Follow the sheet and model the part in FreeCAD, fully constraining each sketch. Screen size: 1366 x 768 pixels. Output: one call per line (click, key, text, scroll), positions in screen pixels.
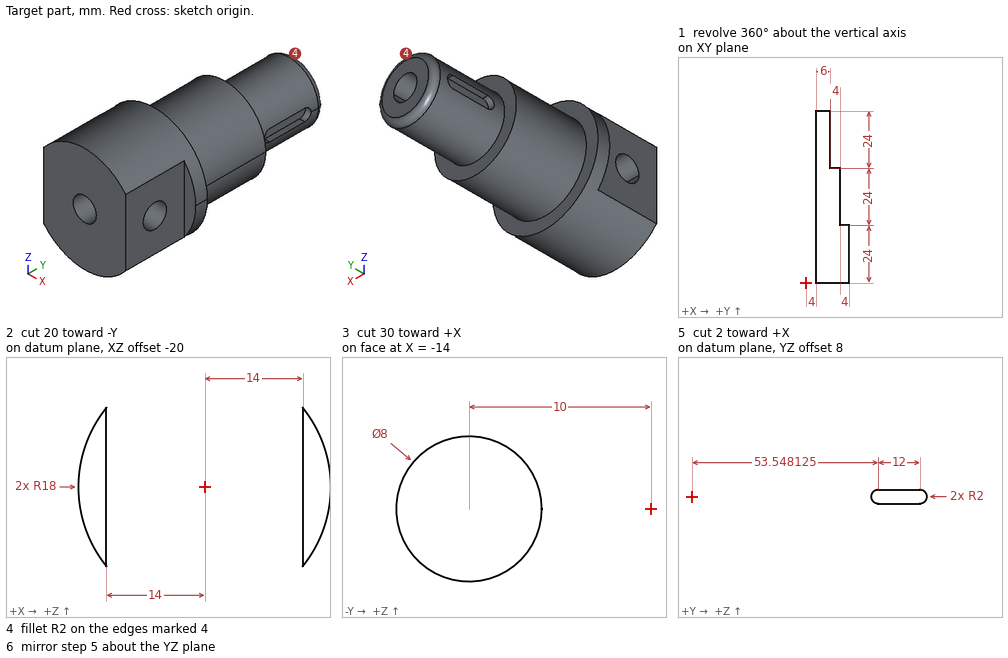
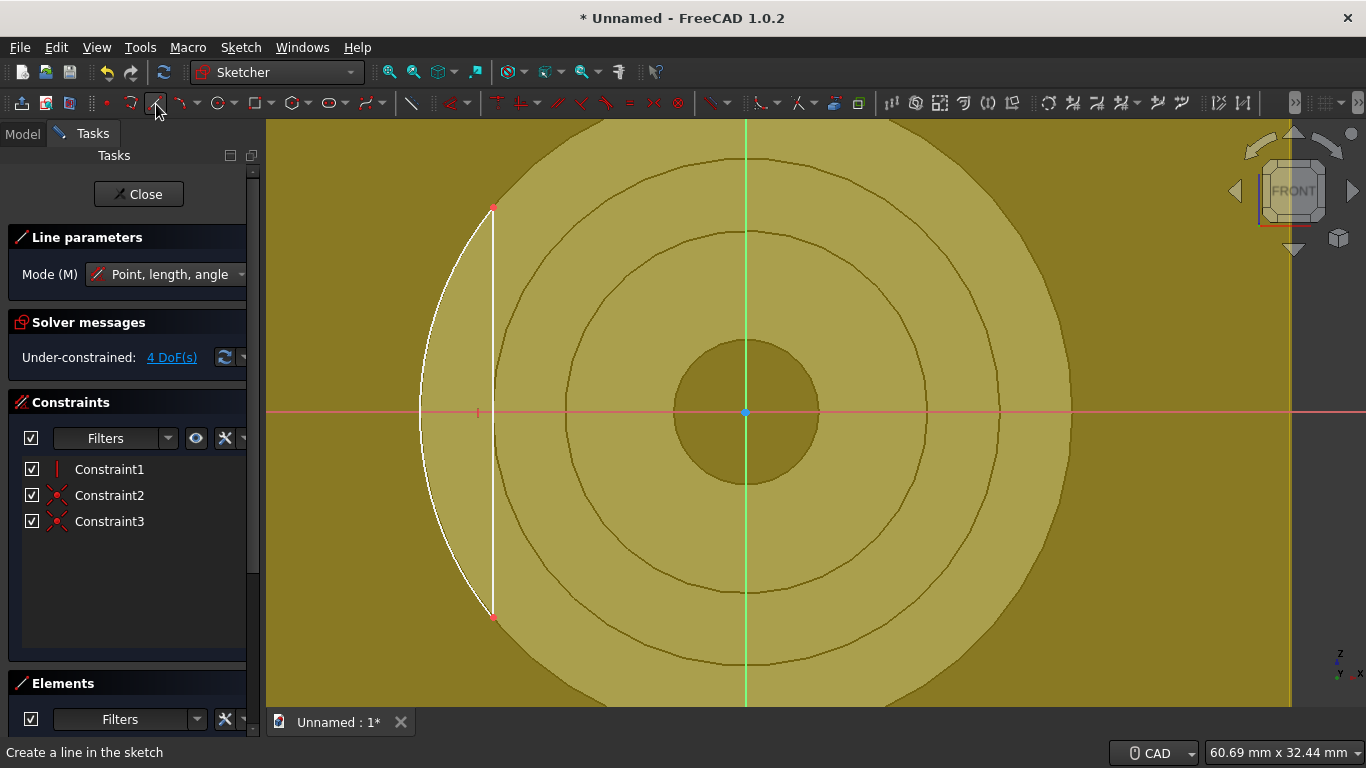
click(1000, 207)
click(1000, 617)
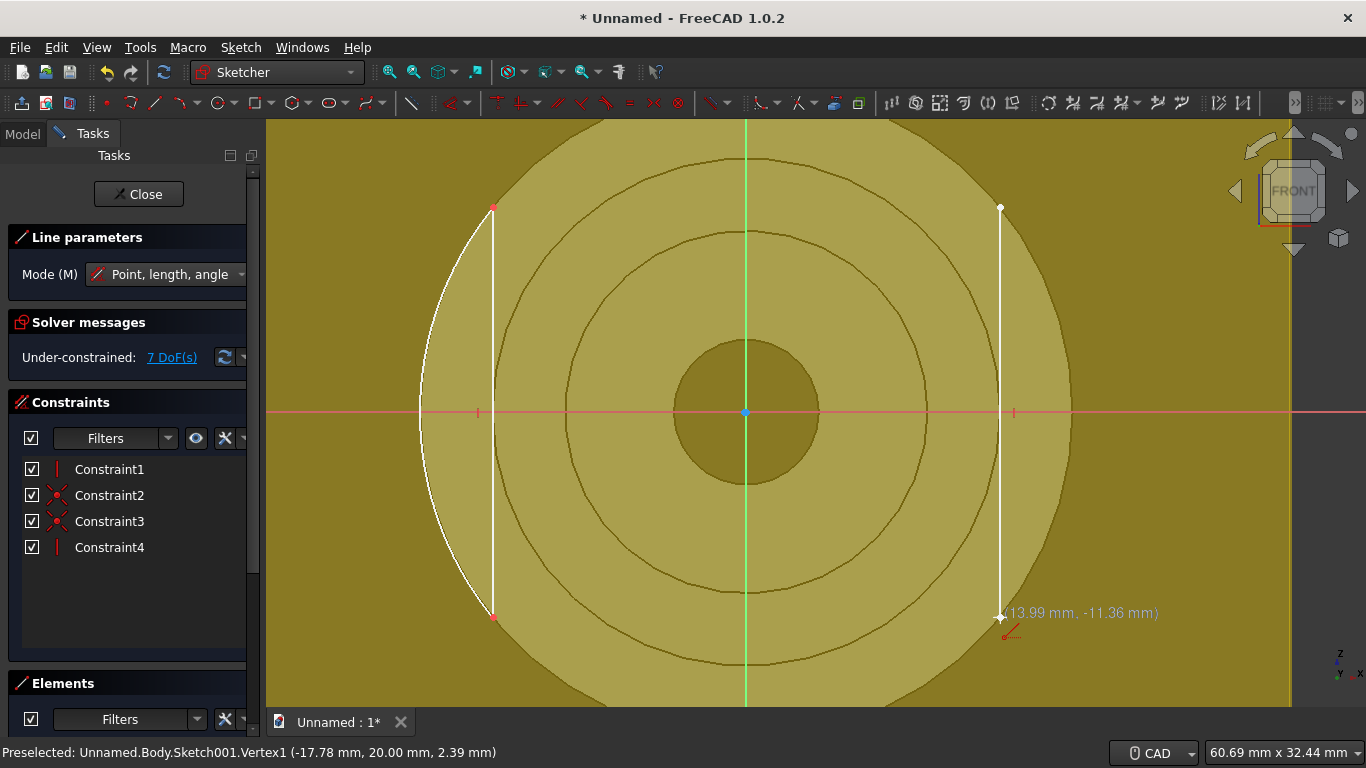
click(180, 104)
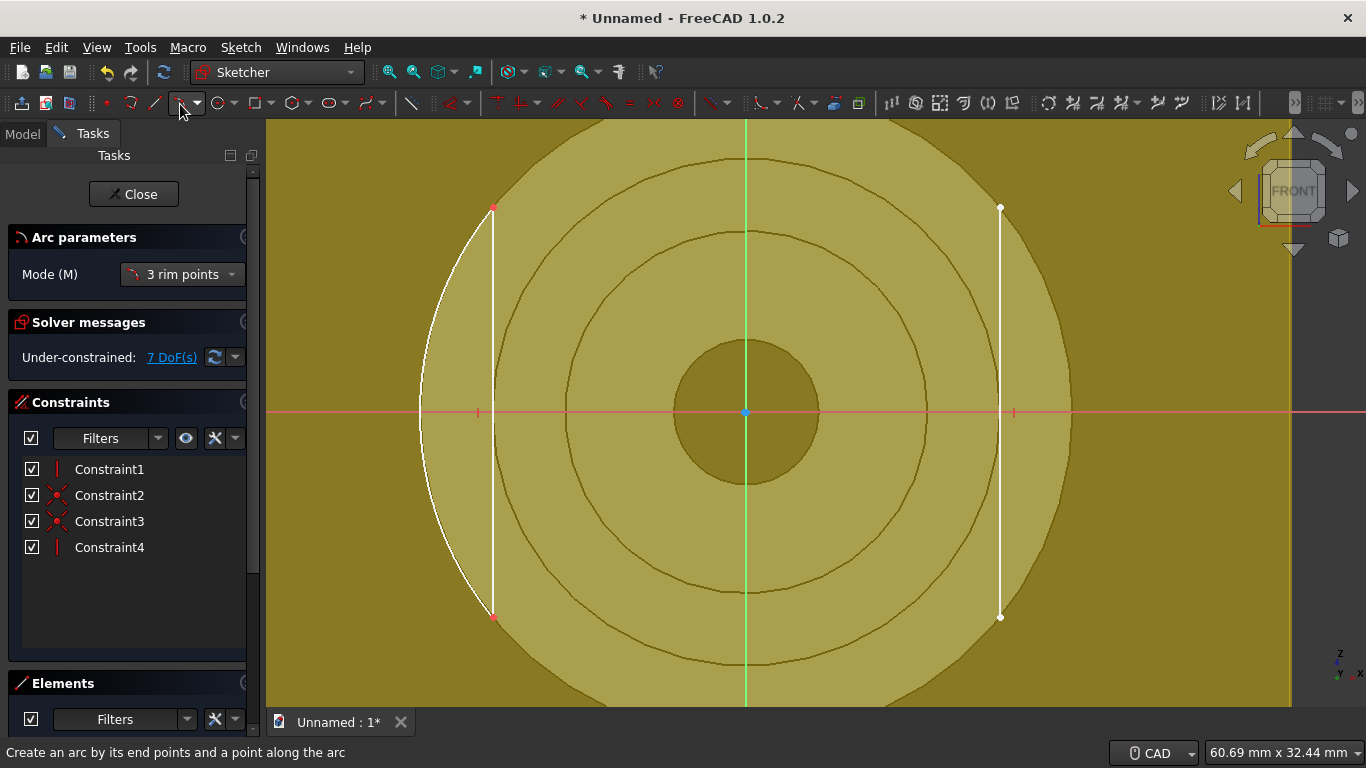
click(1000, 618)
click(1000, 208)
click(1070, 456)
key(Escape)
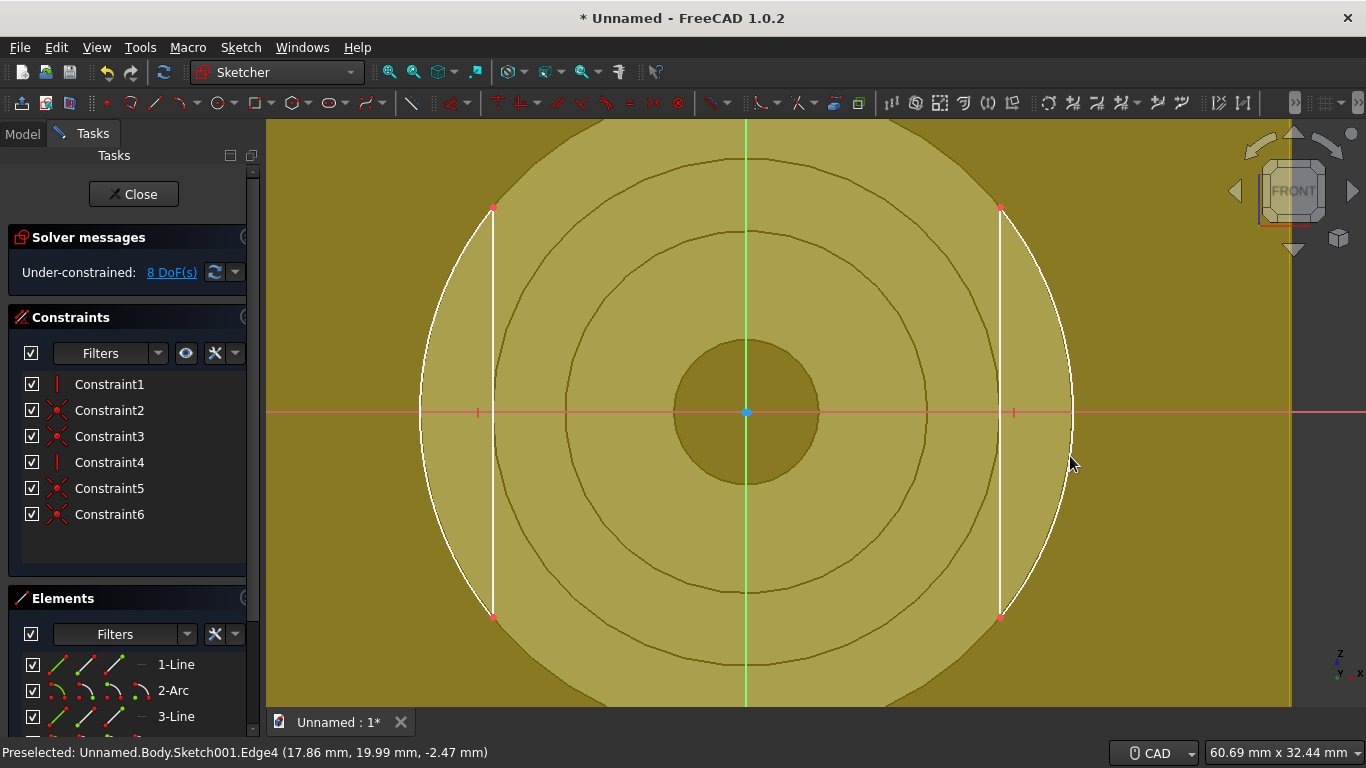
click(432, 325)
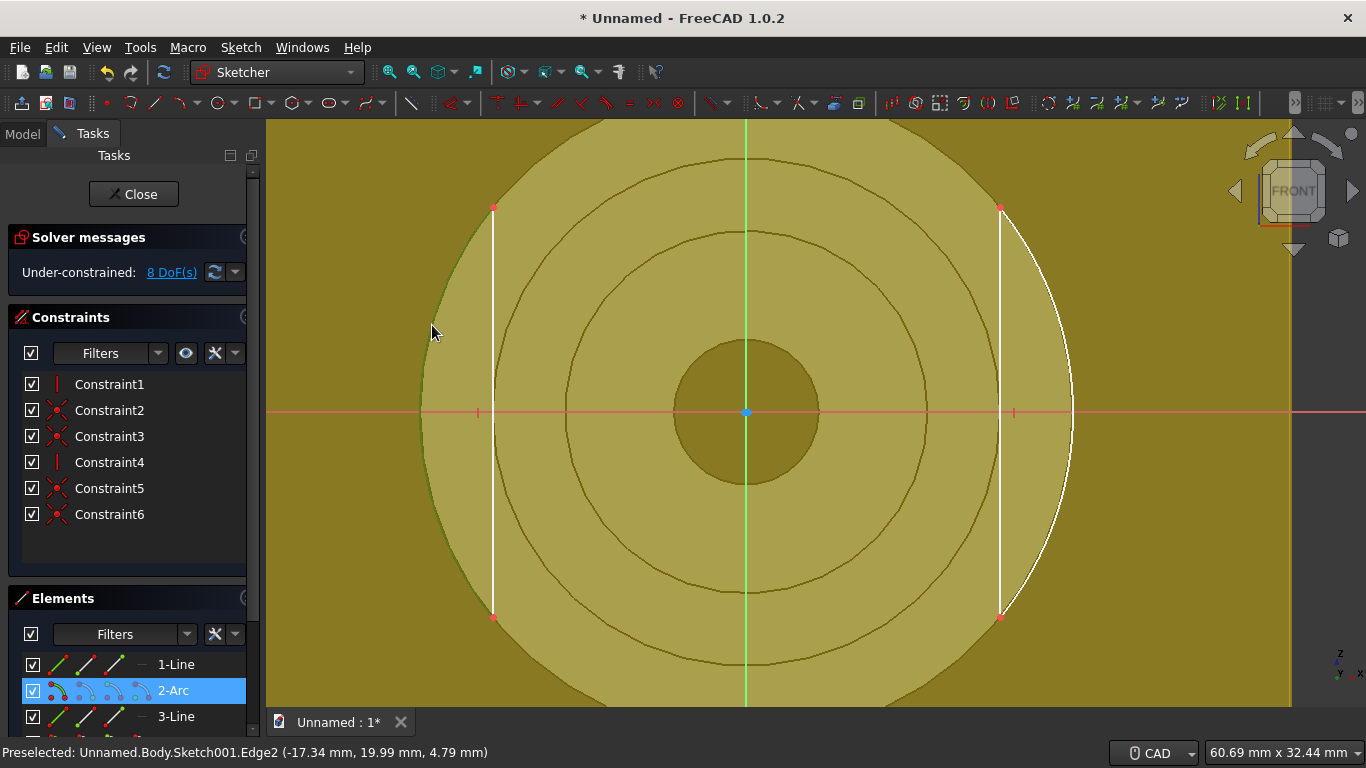
click(1061, 501)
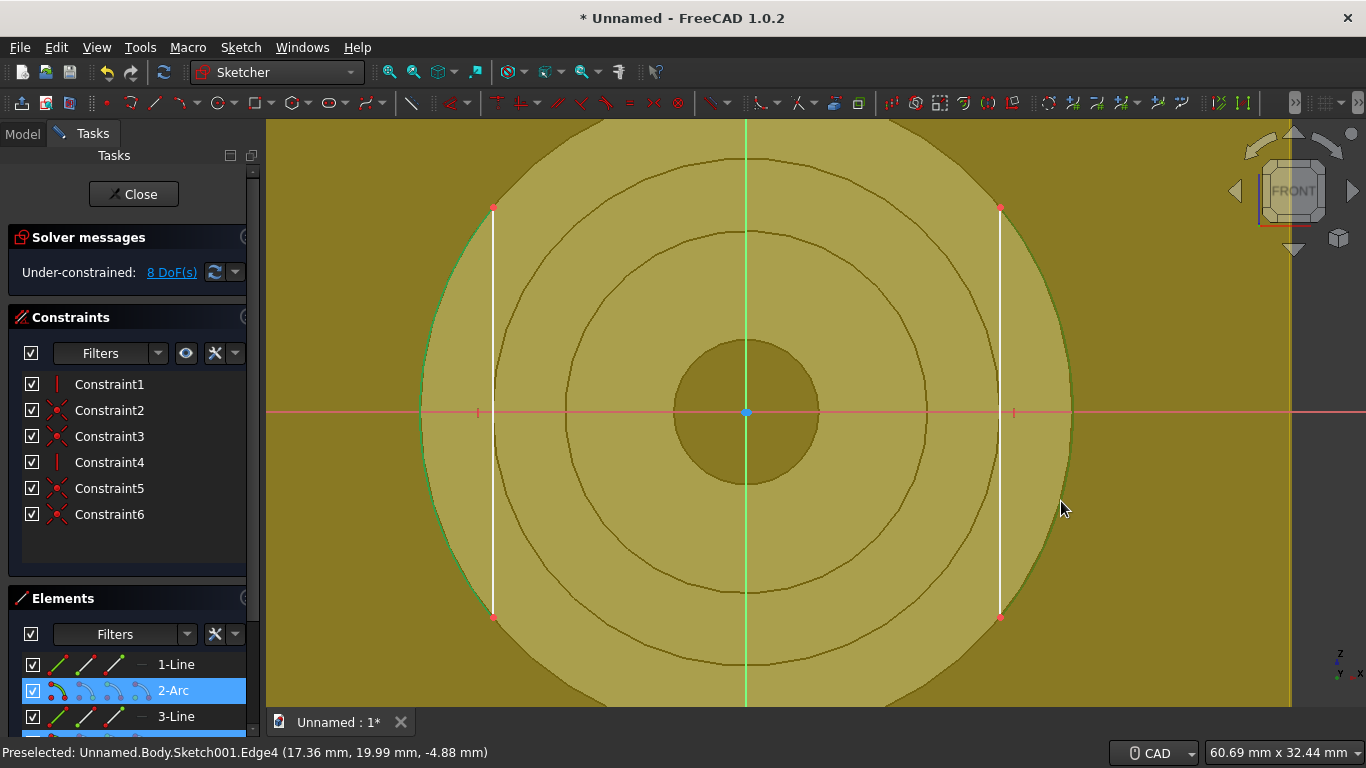
click(498, 104)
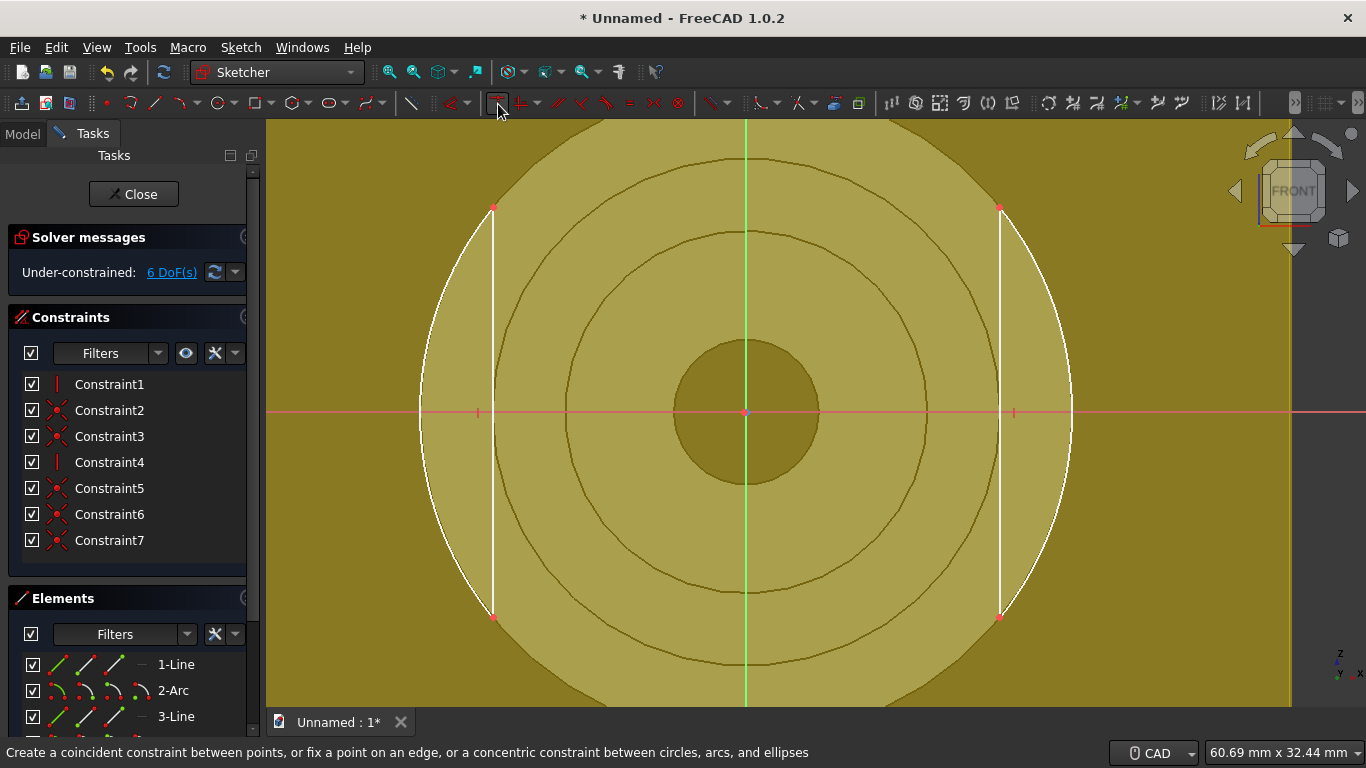
drag(734, 402, 756, 423)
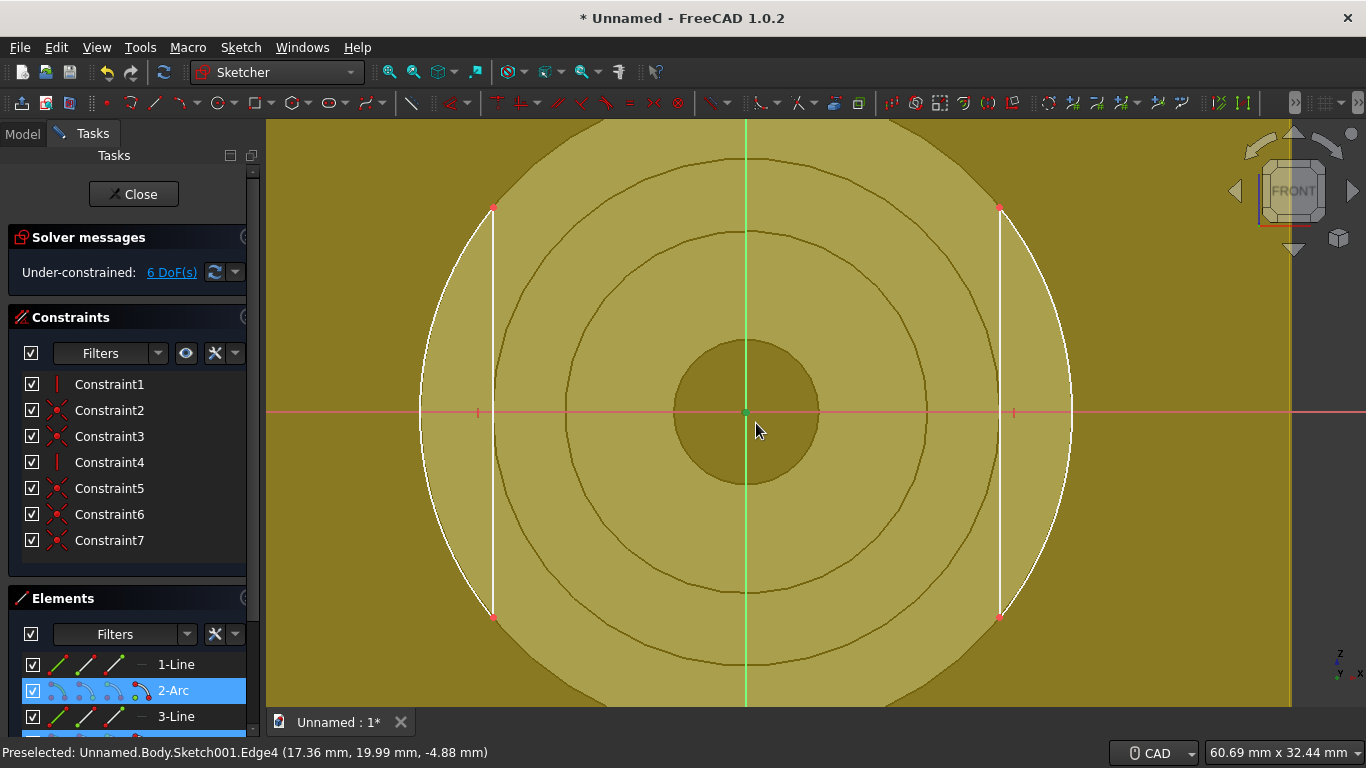
click(498, 104)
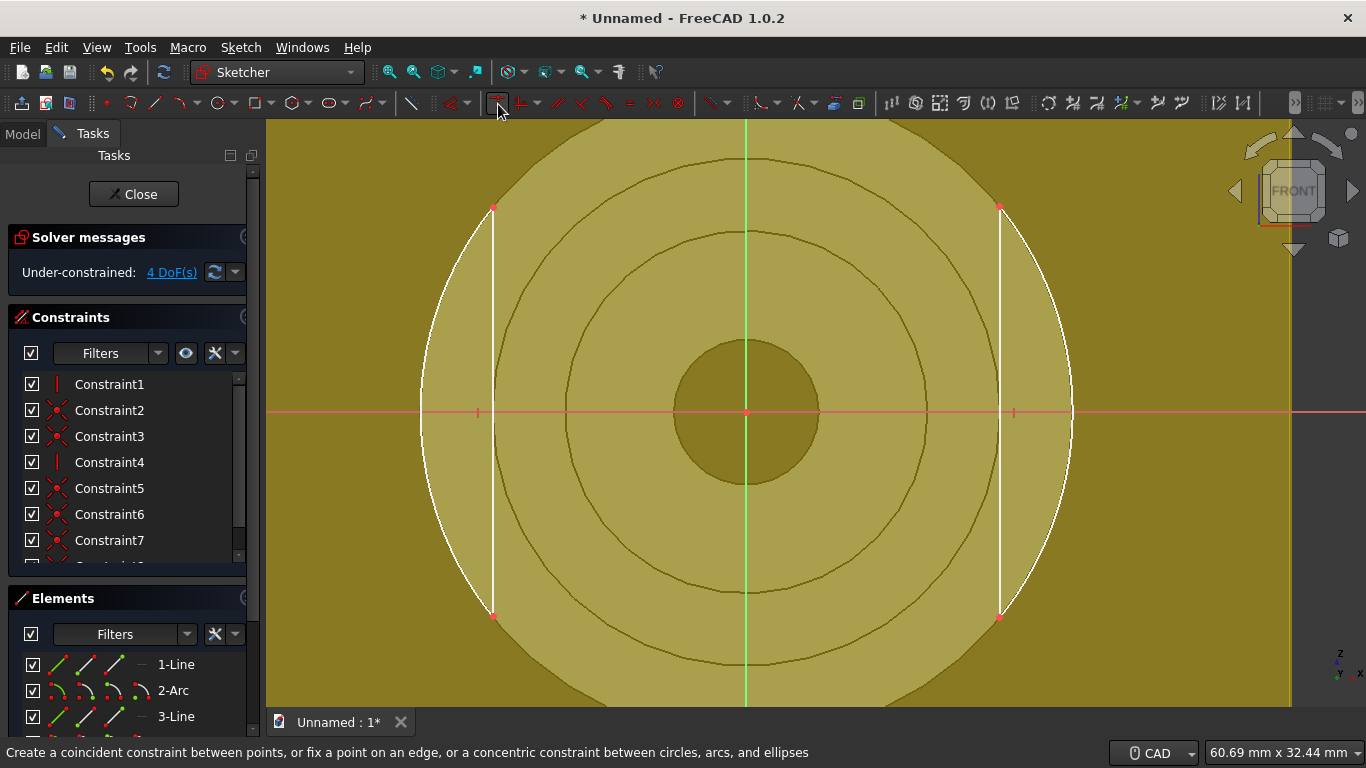
click(433, 325)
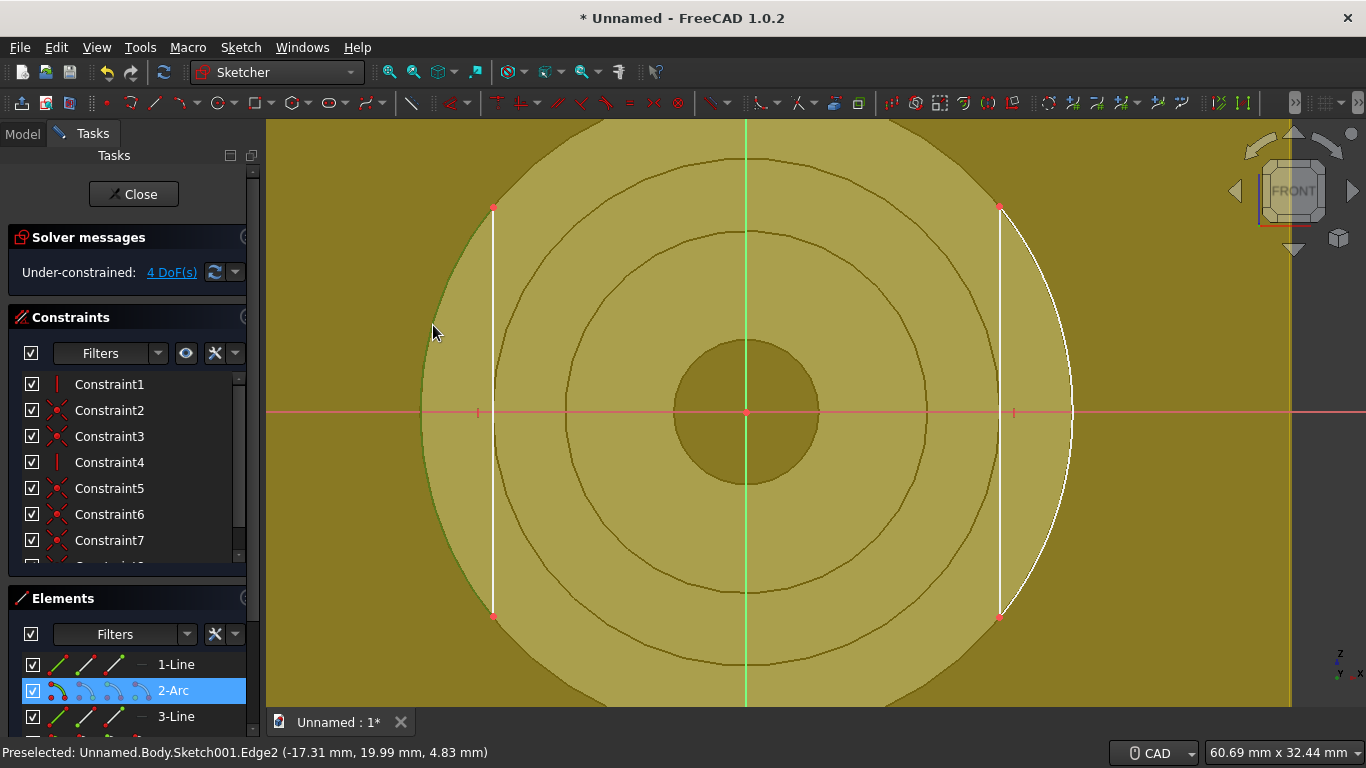
click(1061, 500)